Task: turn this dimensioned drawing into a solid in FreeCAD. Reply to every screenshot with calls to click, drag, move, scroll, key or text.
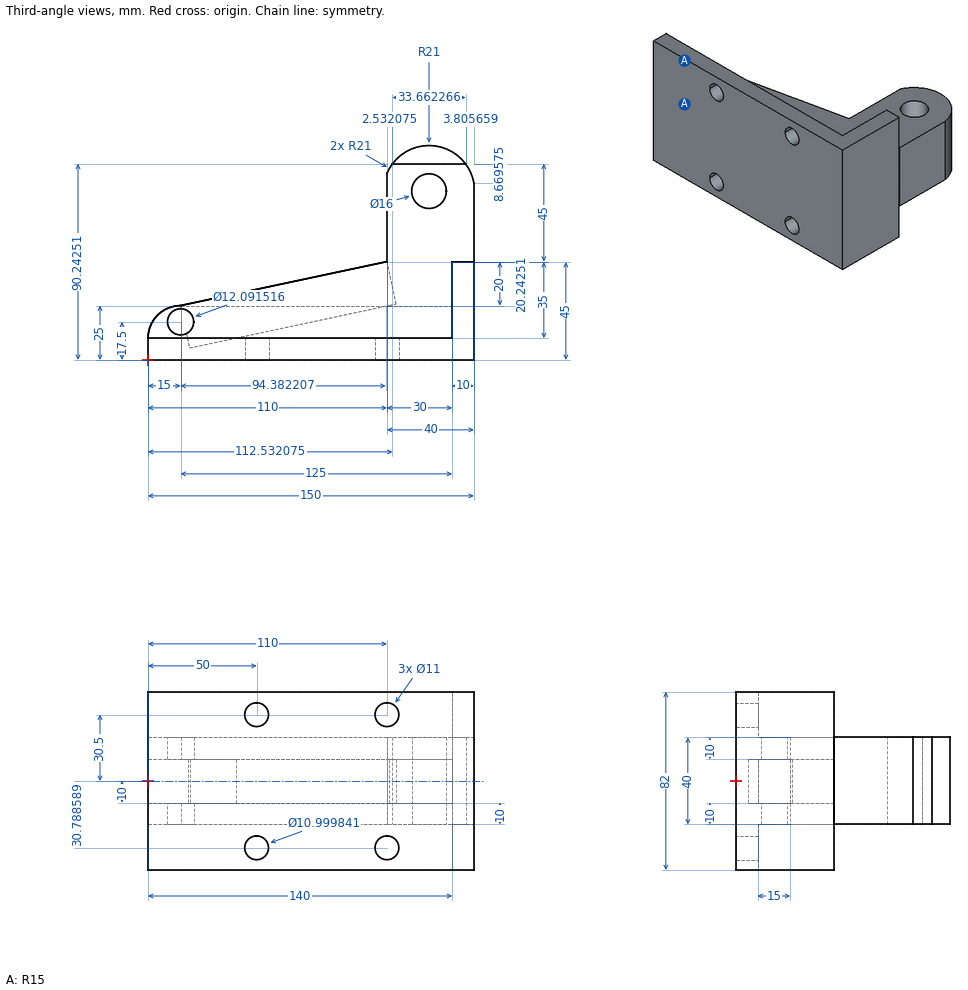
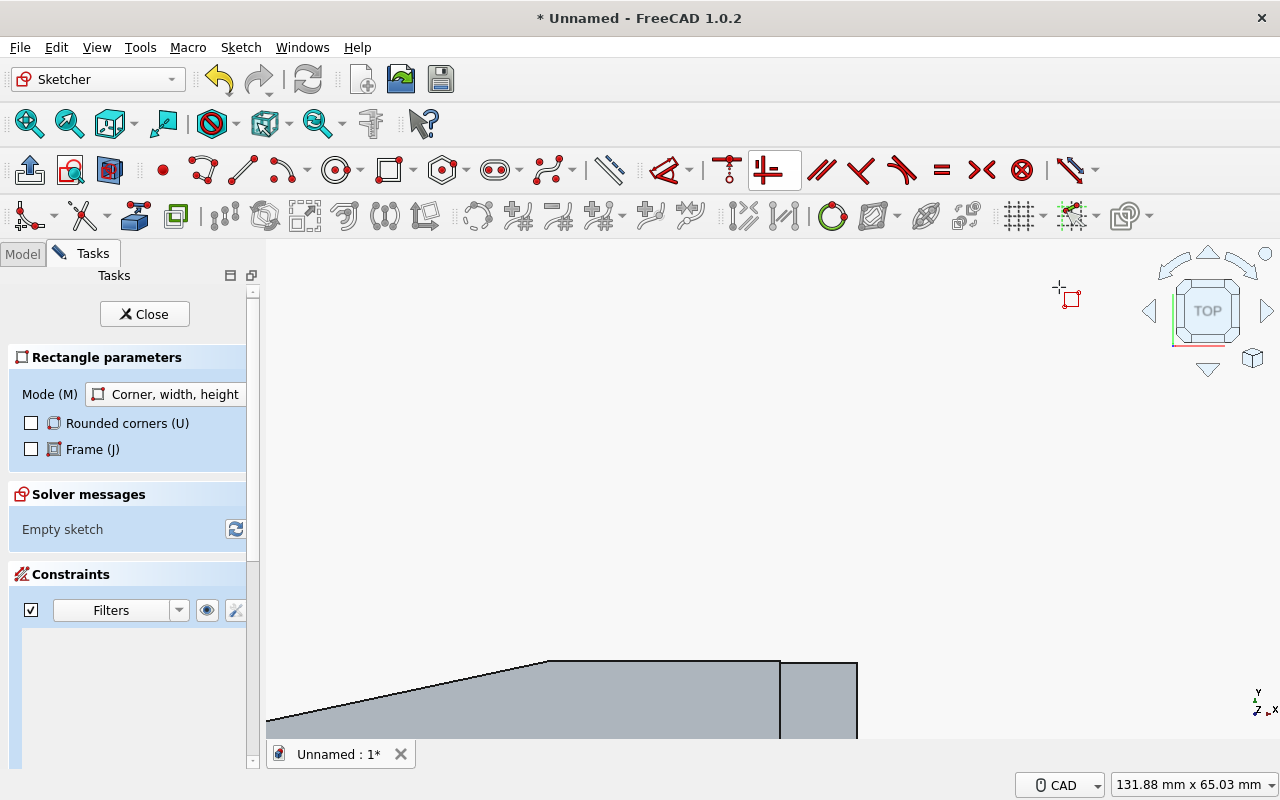
click(549, 315)
move(857, 661)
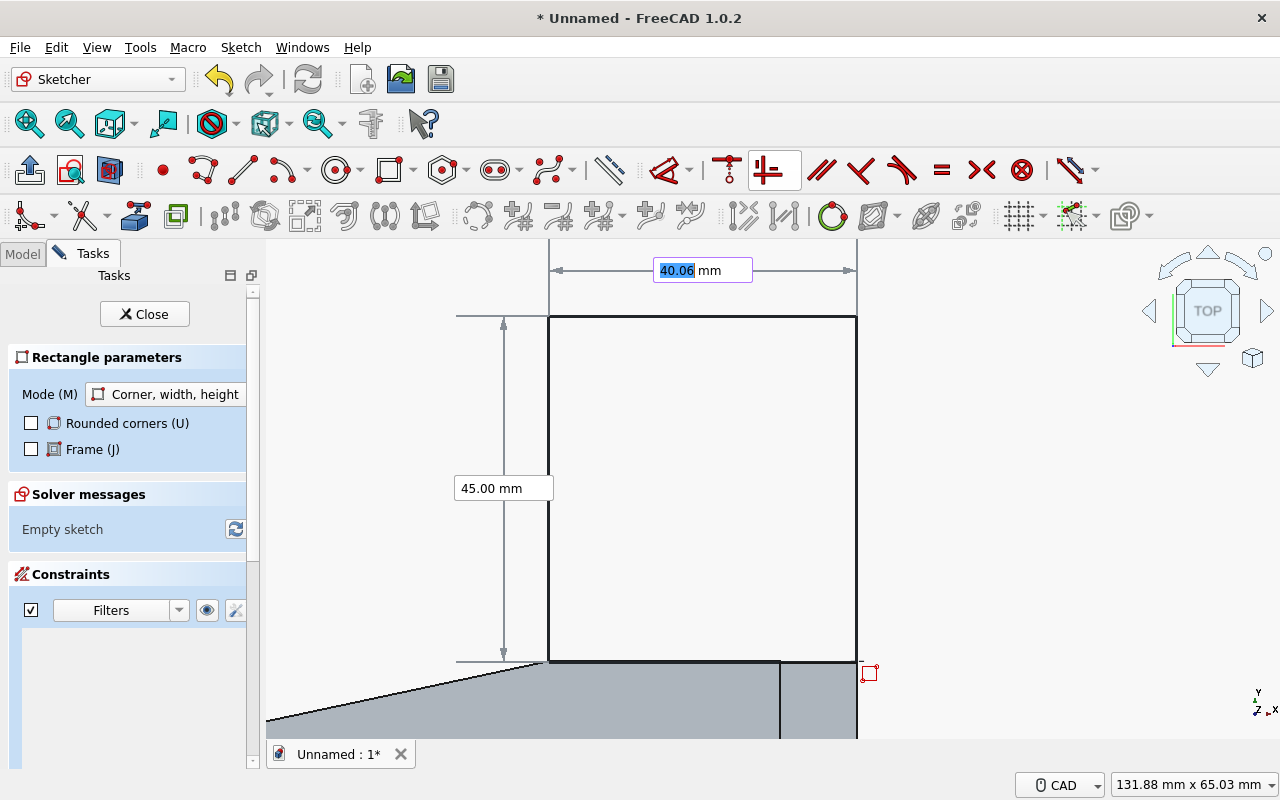
text(40)
key(Tab)
text(45)
key(Return)
key(Escape)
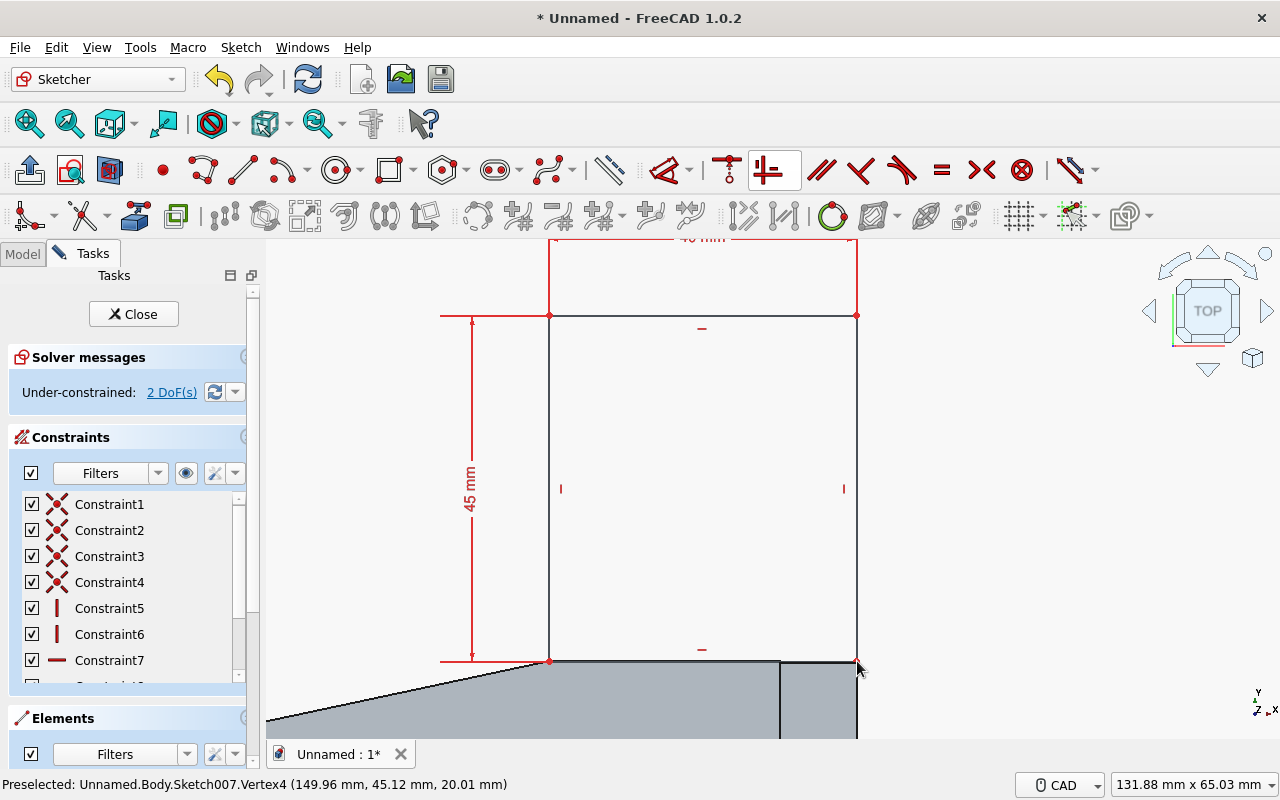
key(d)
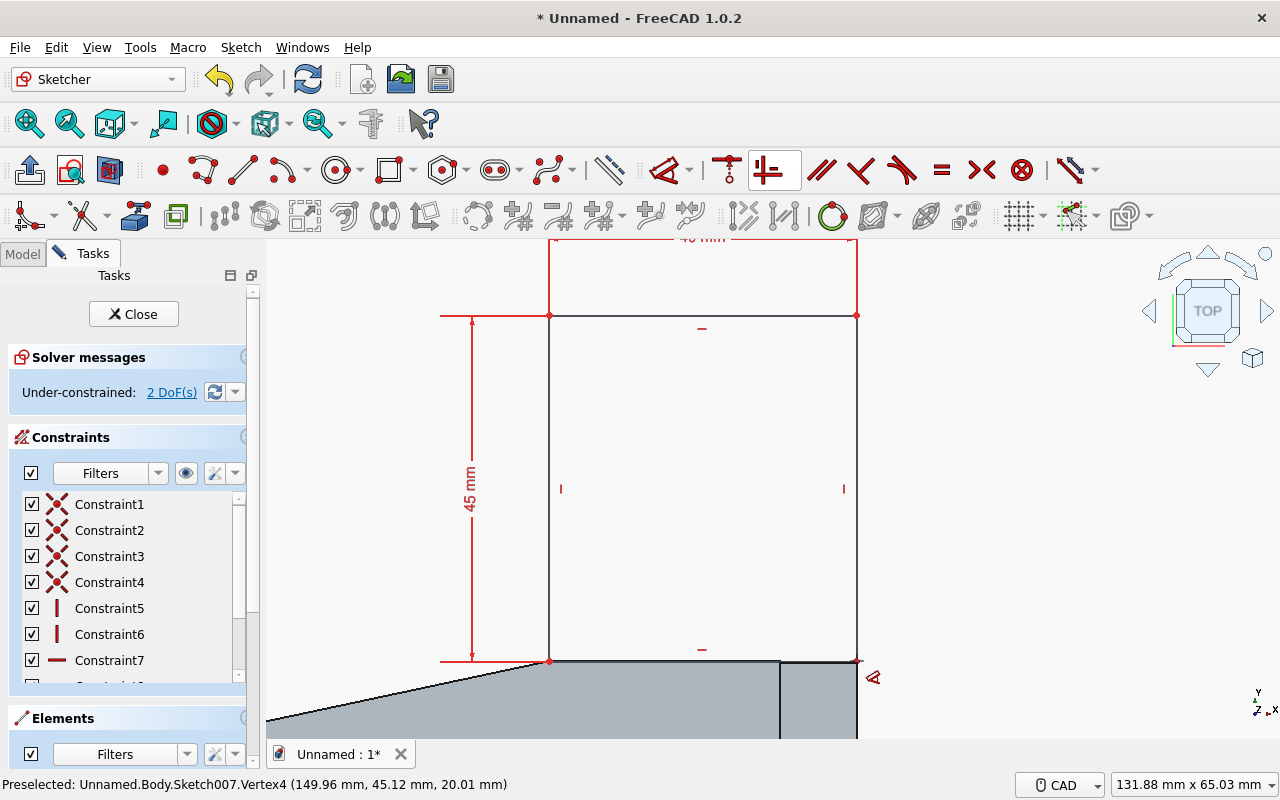
click(549, 316)
click(422, 282)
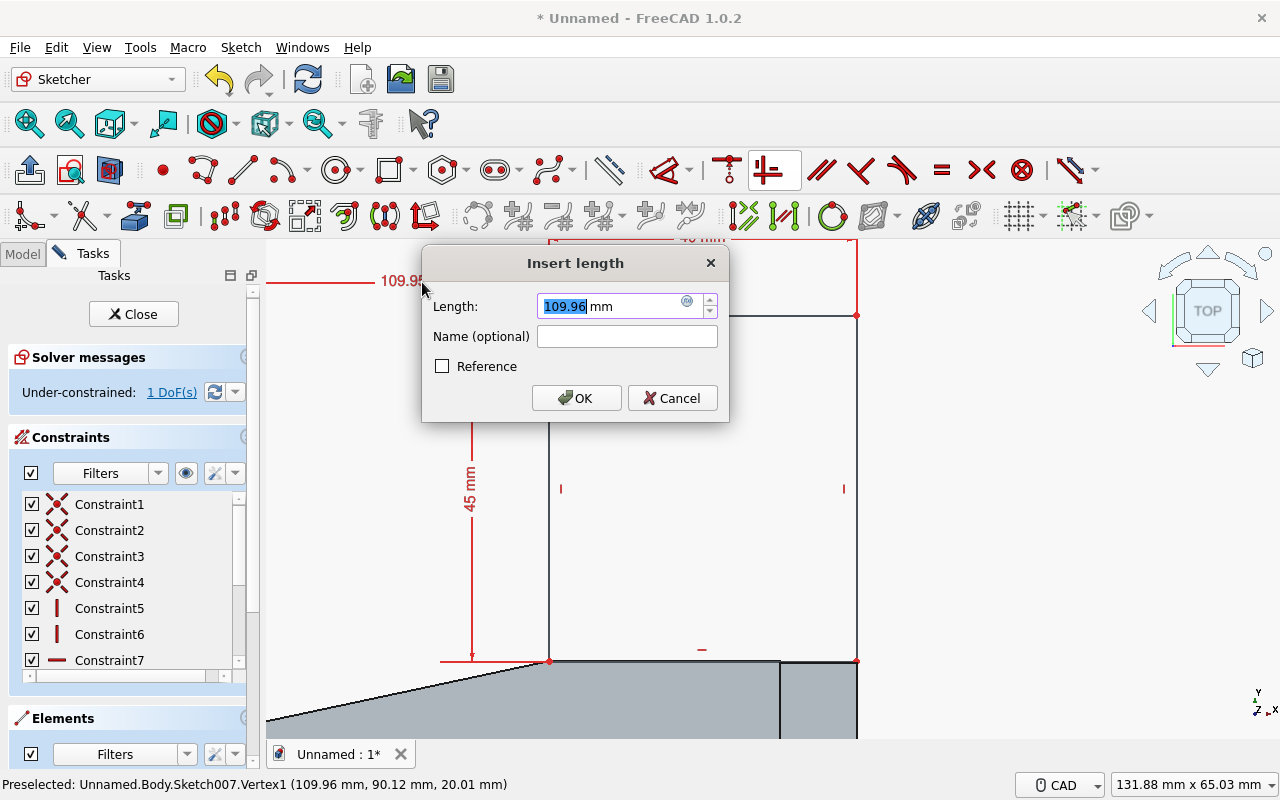
text(110)
key(Return)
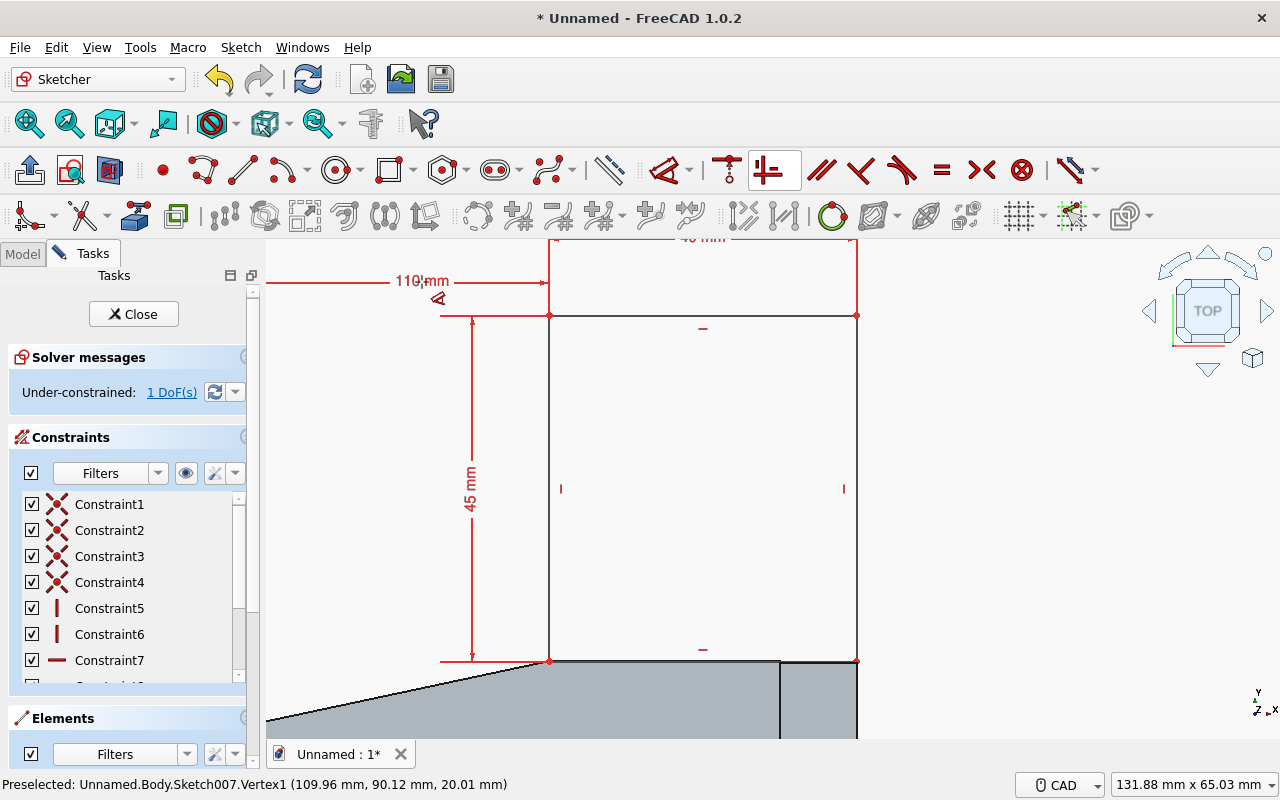
click(549, 316)
click(583, 513)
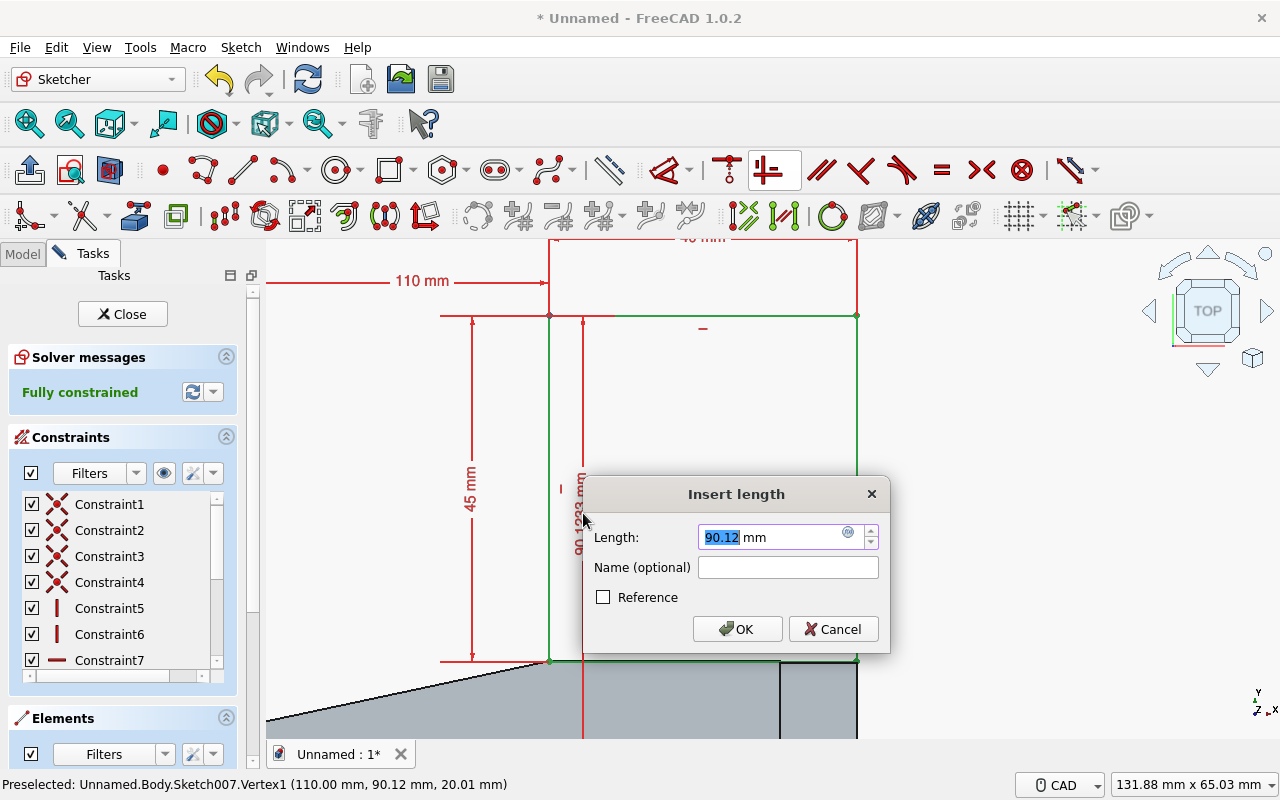
text(90.24251)
key(Return)
key(Escape)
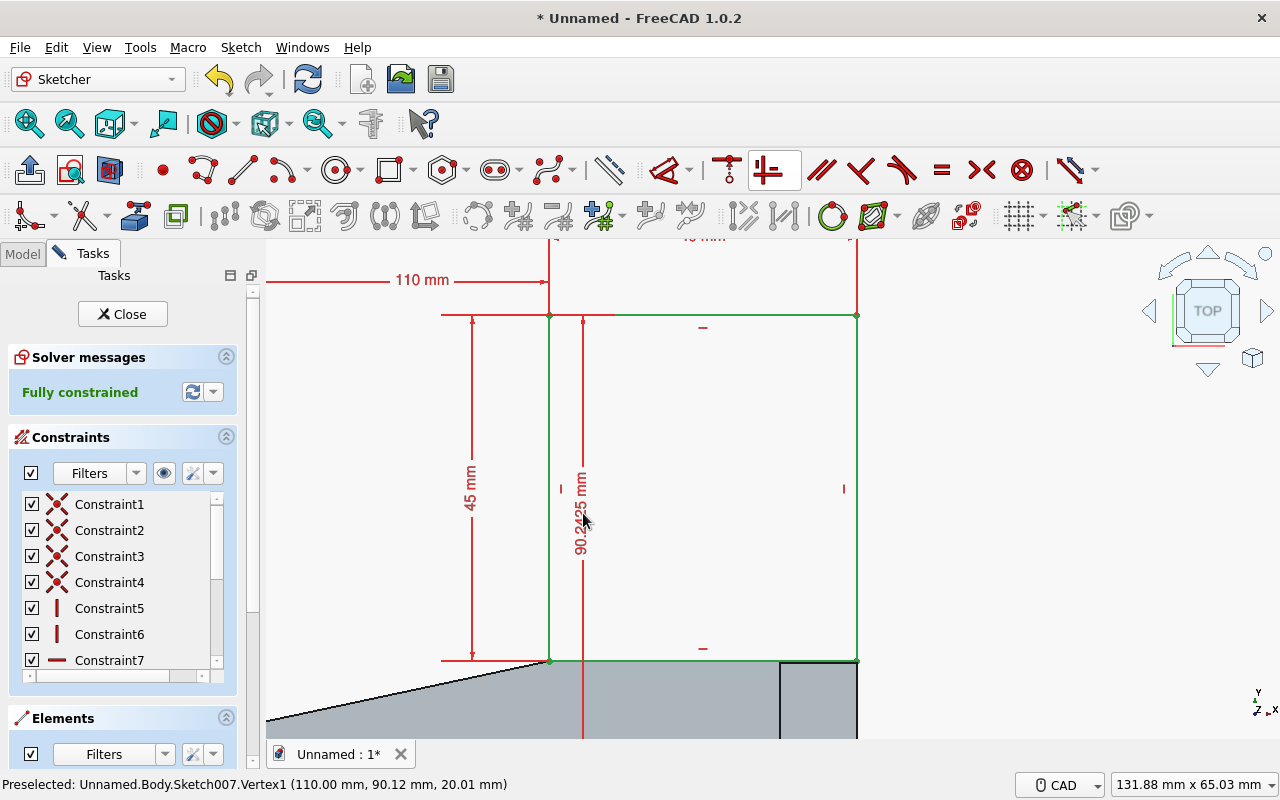
click(123, 314)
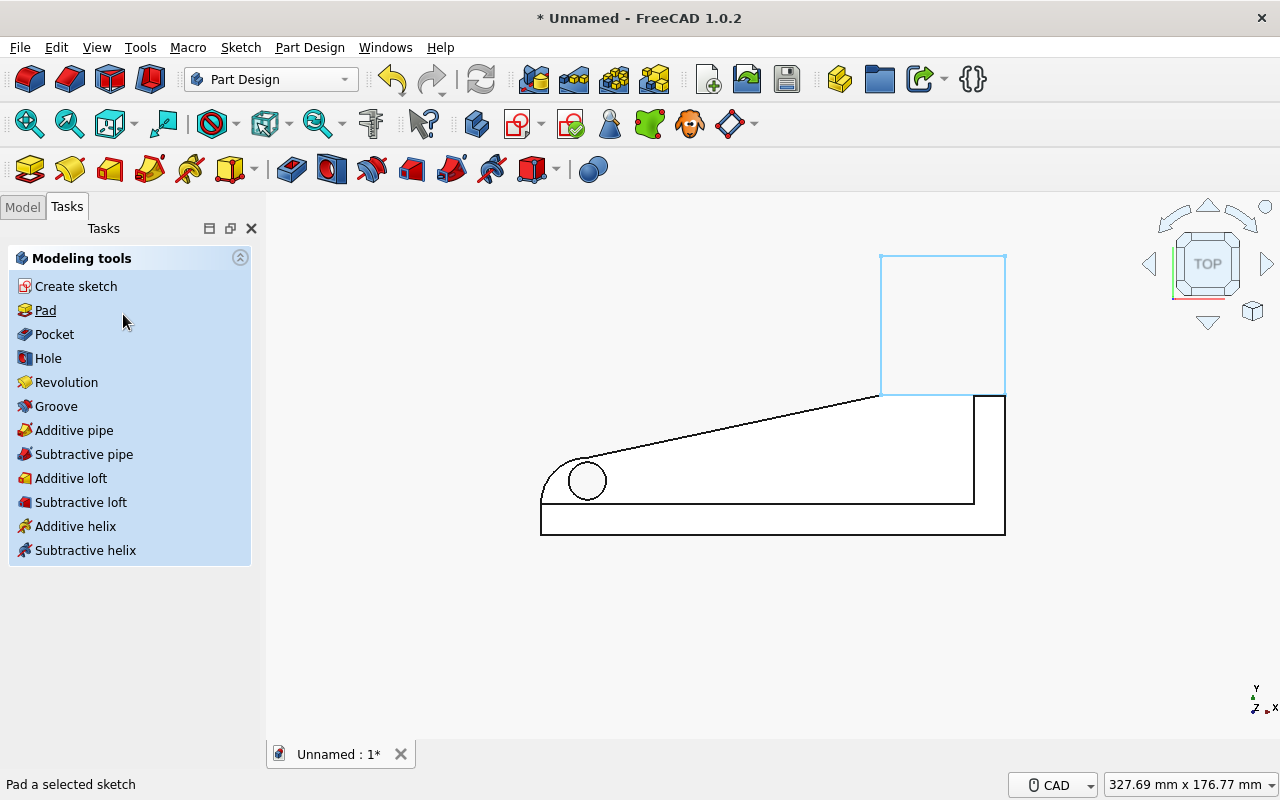
click(30, 170)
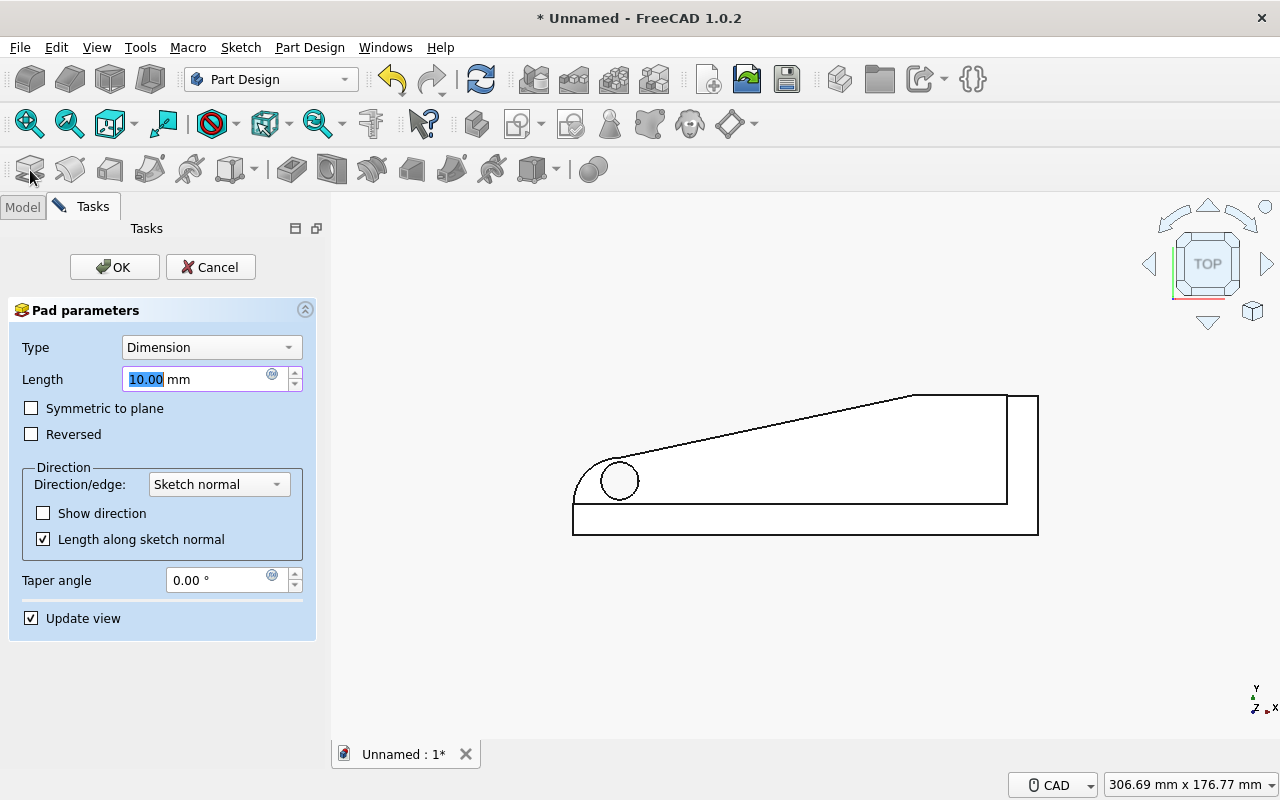
text(40)
key(Tab)